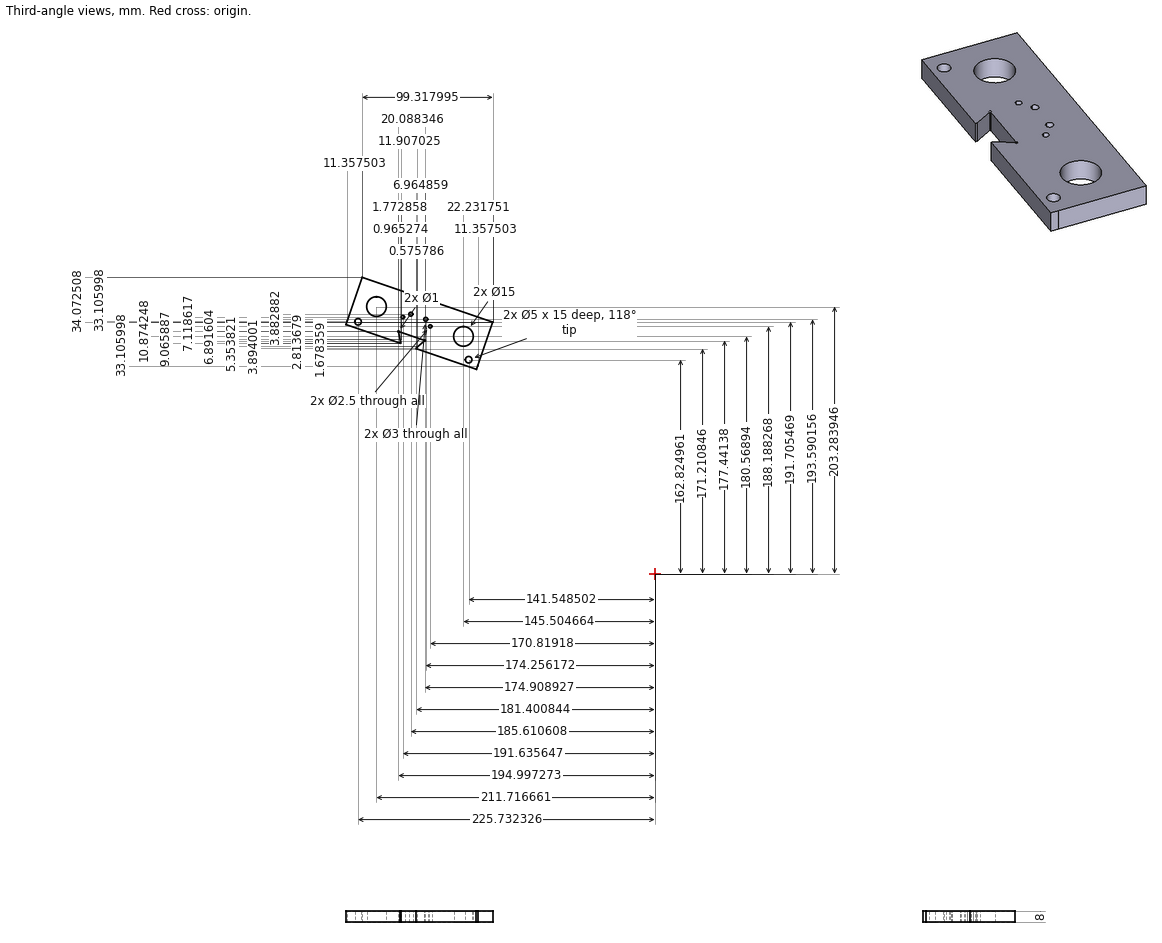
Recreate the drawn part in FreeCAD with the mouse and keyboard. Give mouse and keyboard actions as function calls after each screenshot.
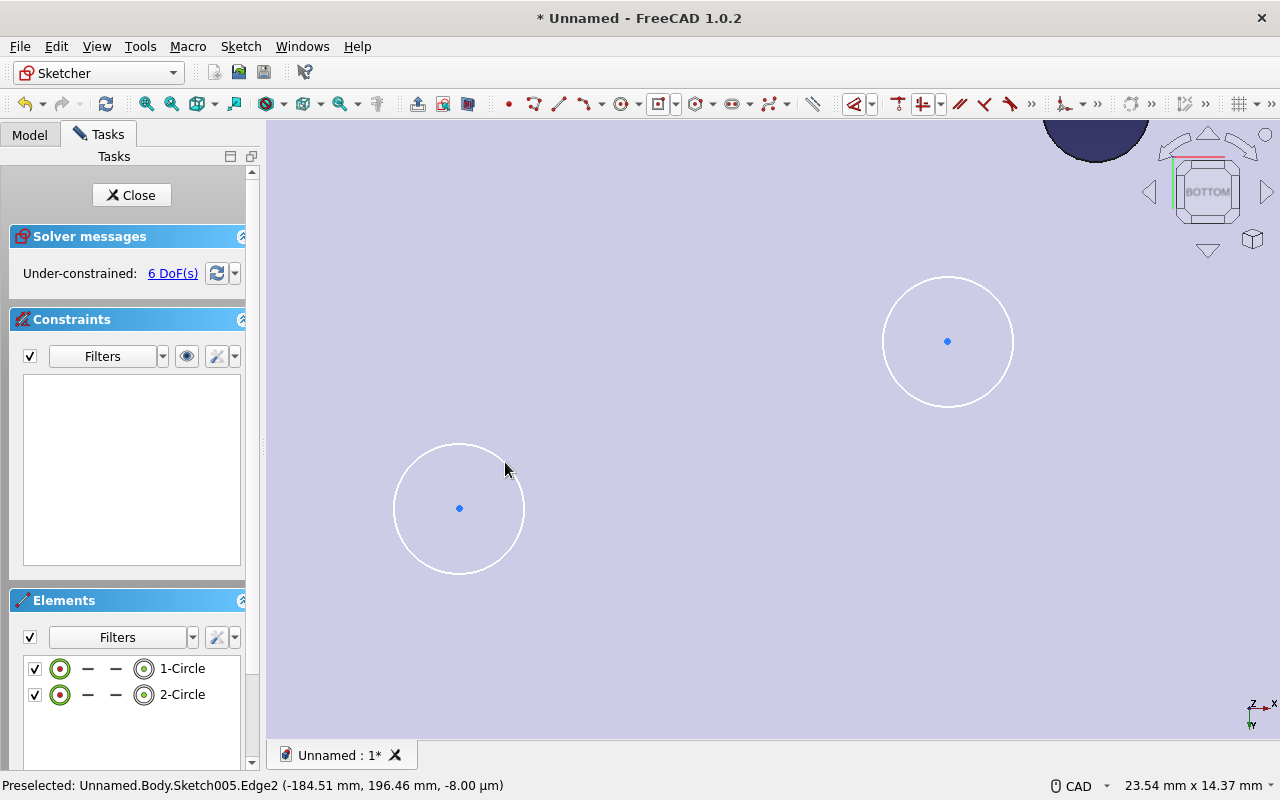
click(994, 296)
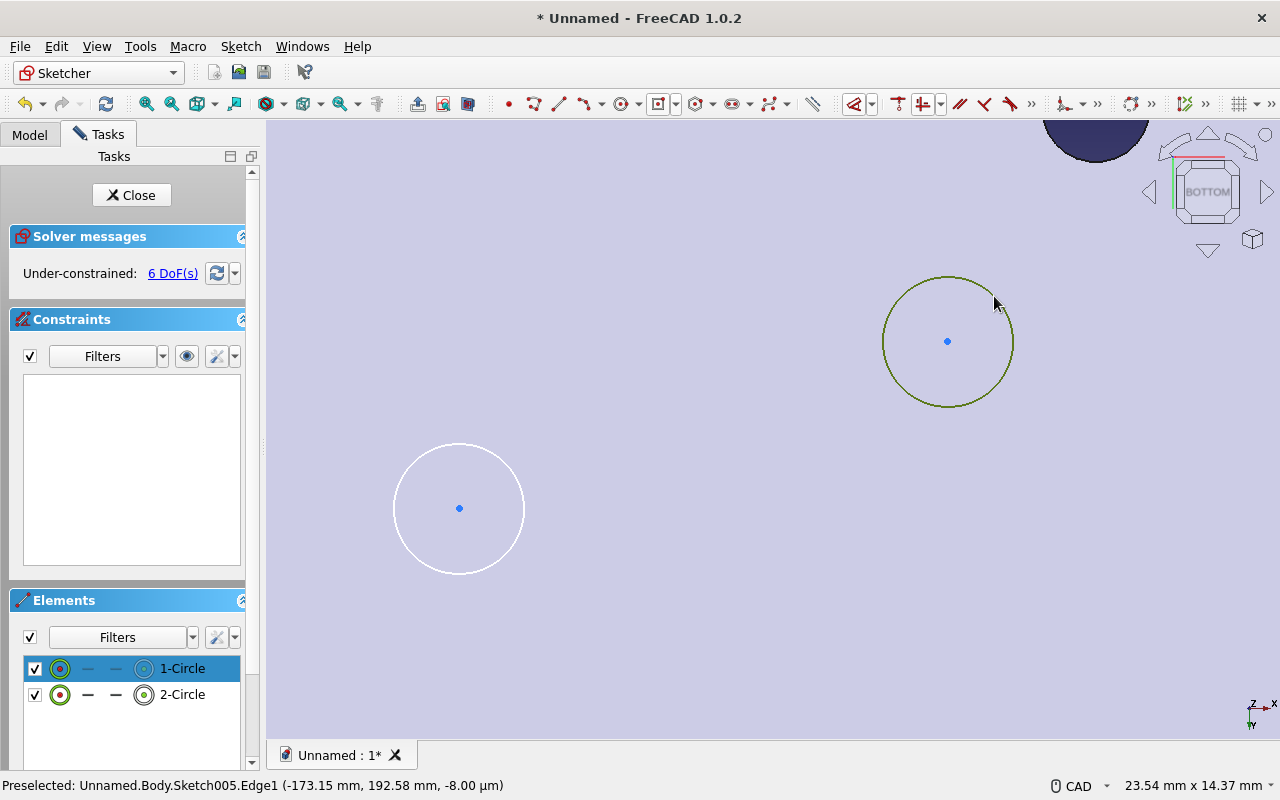
click(505, 463)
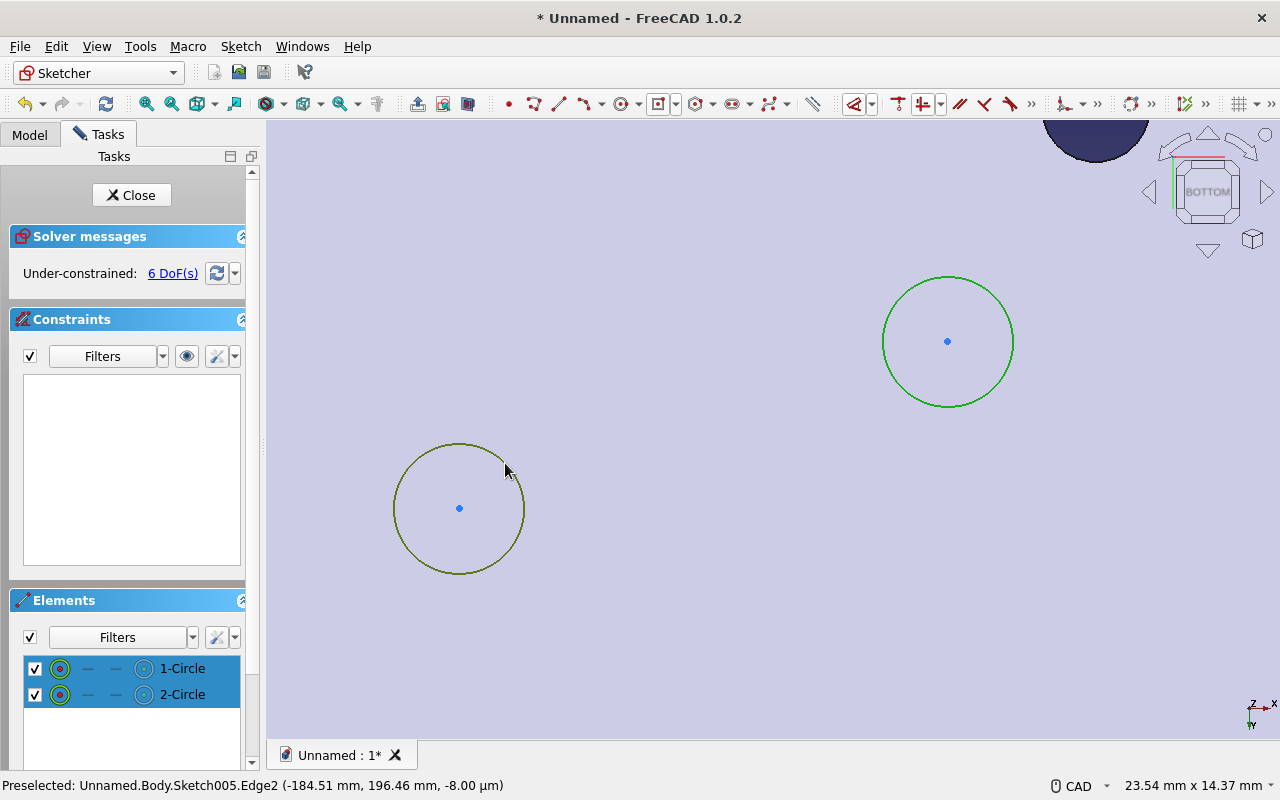
key(e)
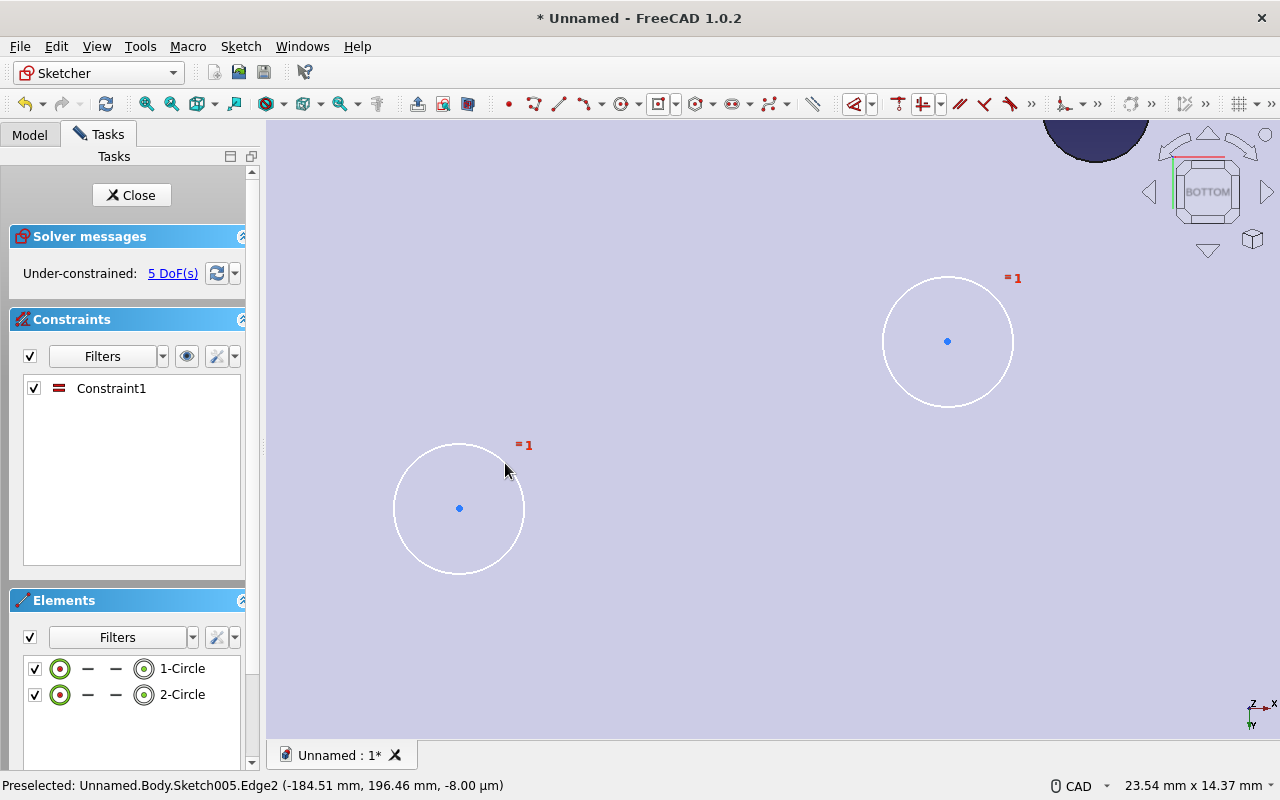
click(994, 296)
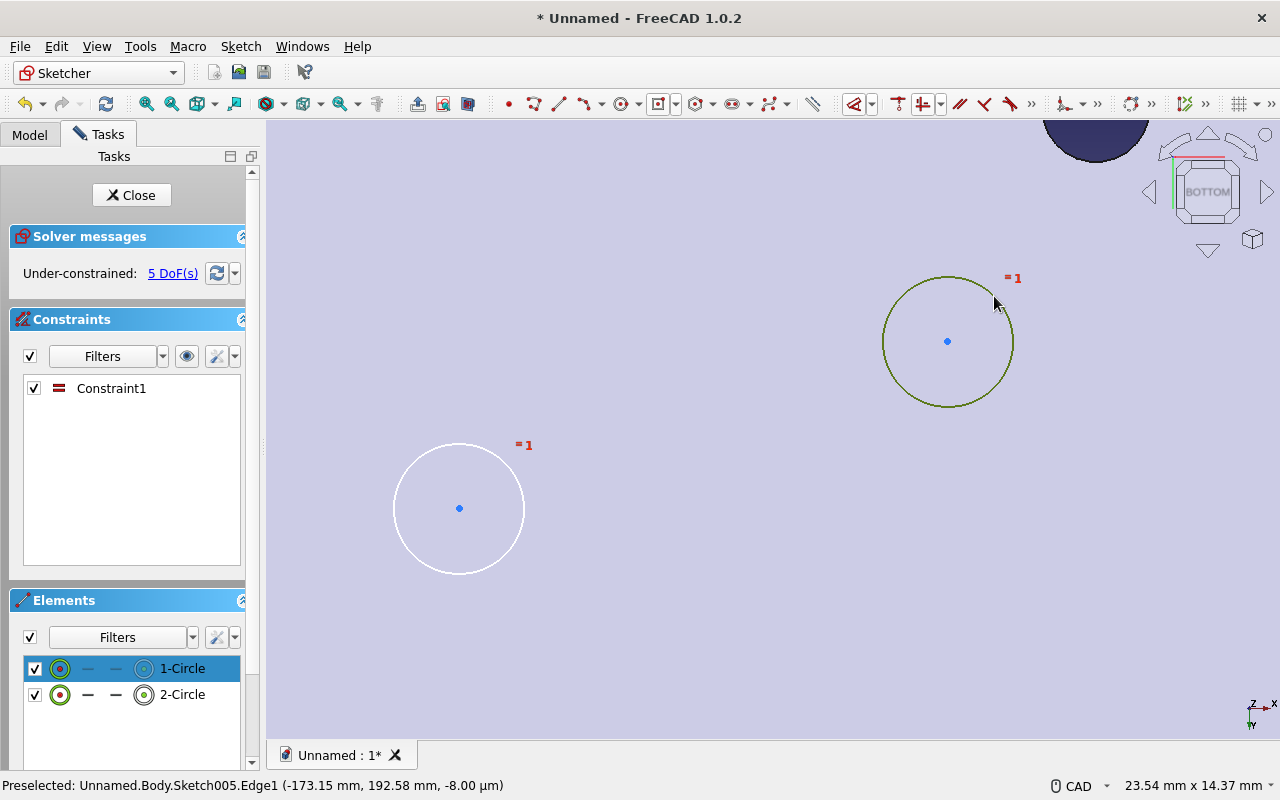
key(k)
key(o)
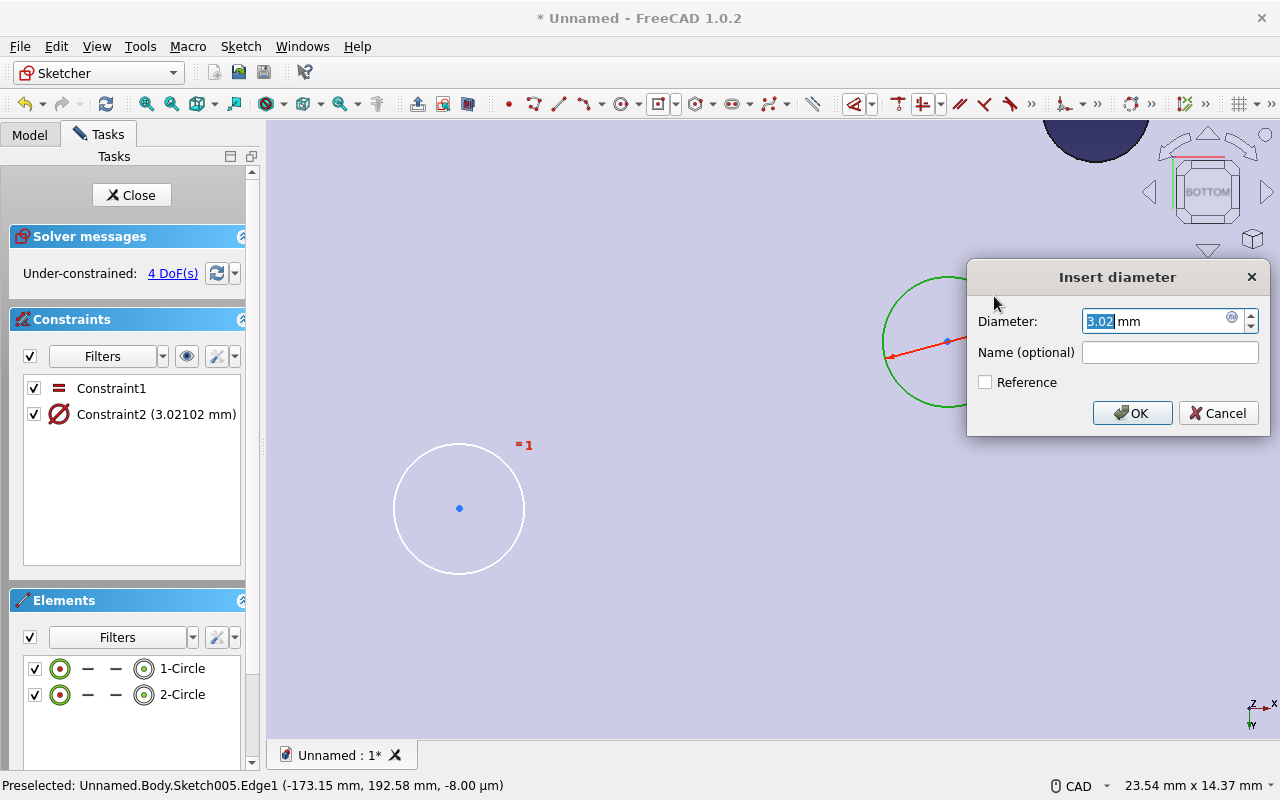
text(3)
key(Return)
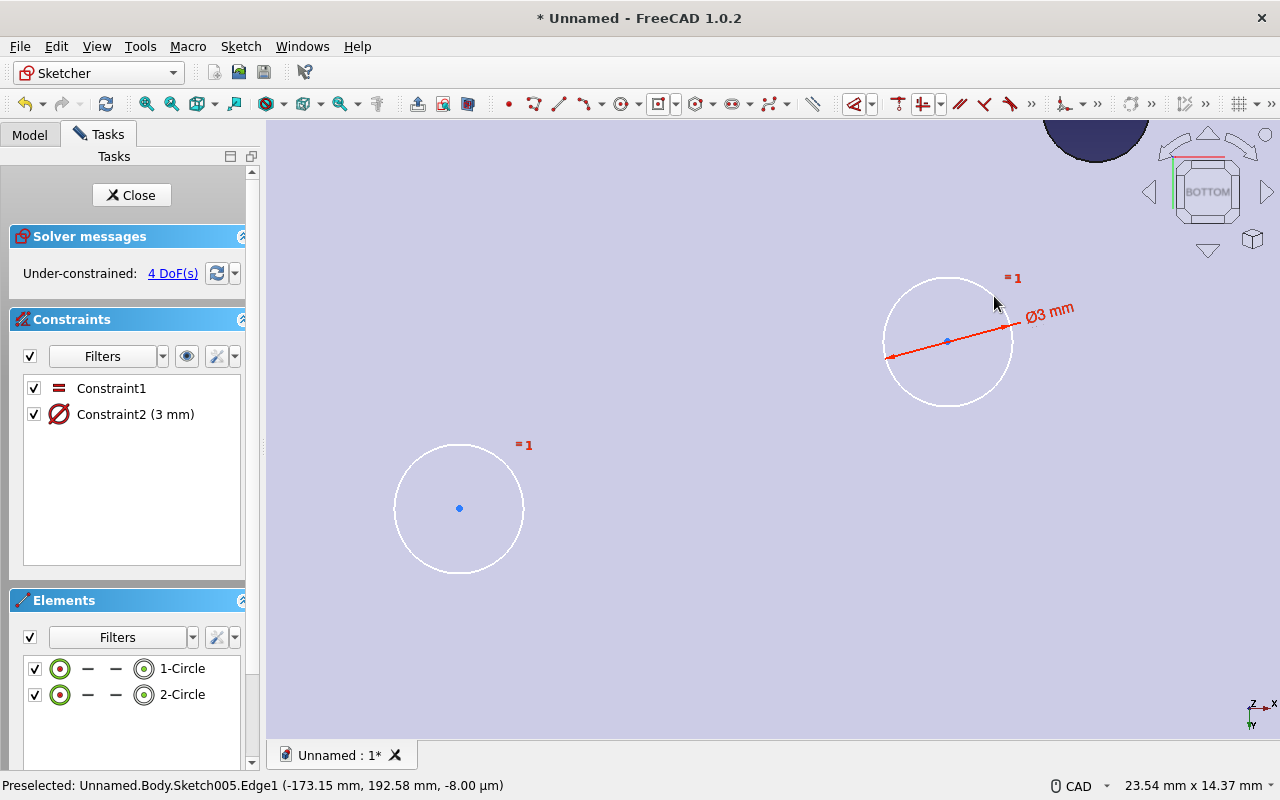
click(948, 342)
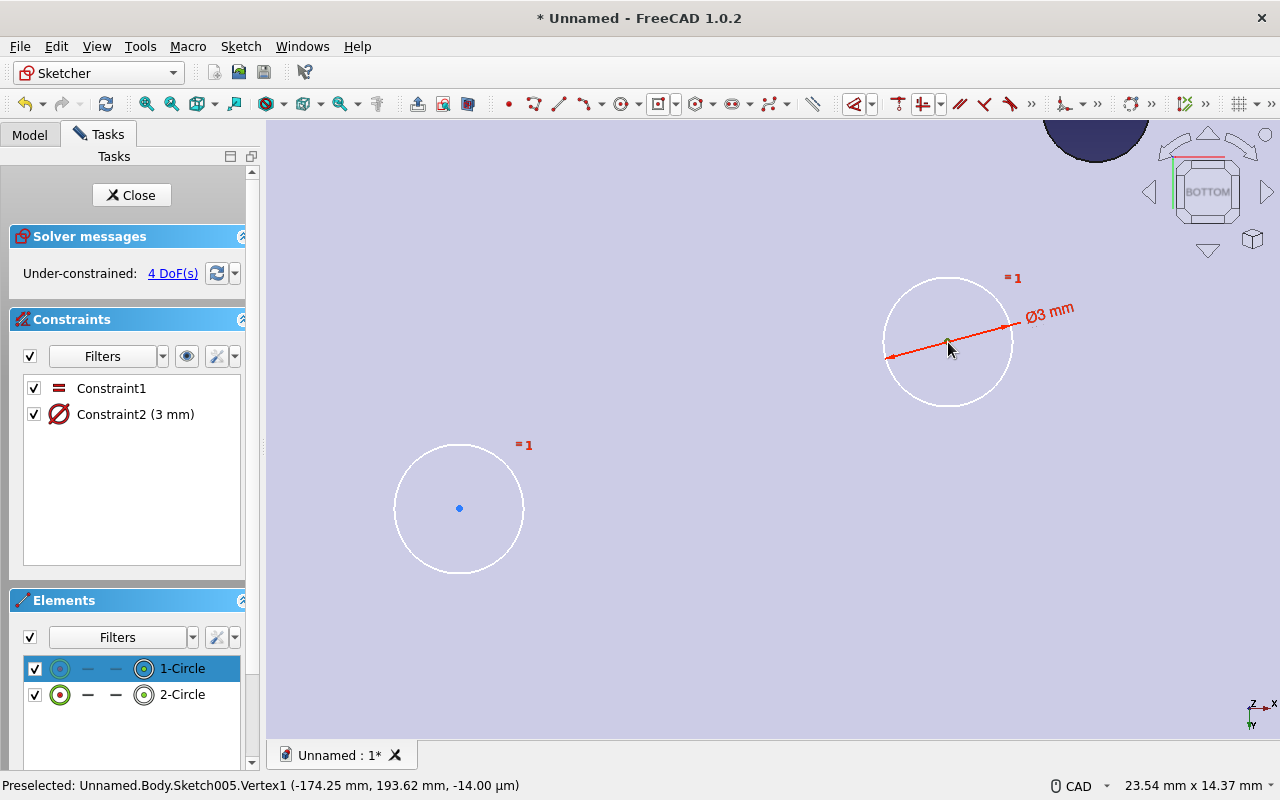
click(459, 509)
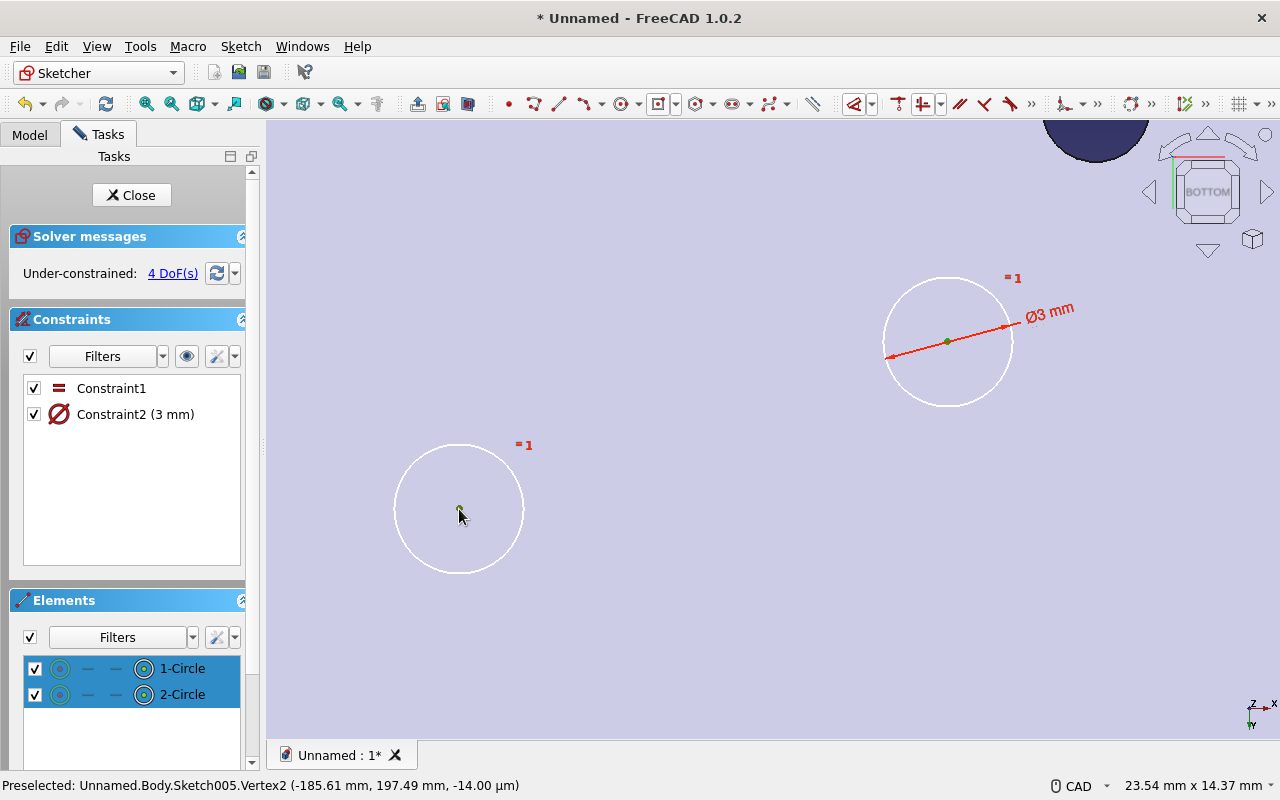
click(872, 104)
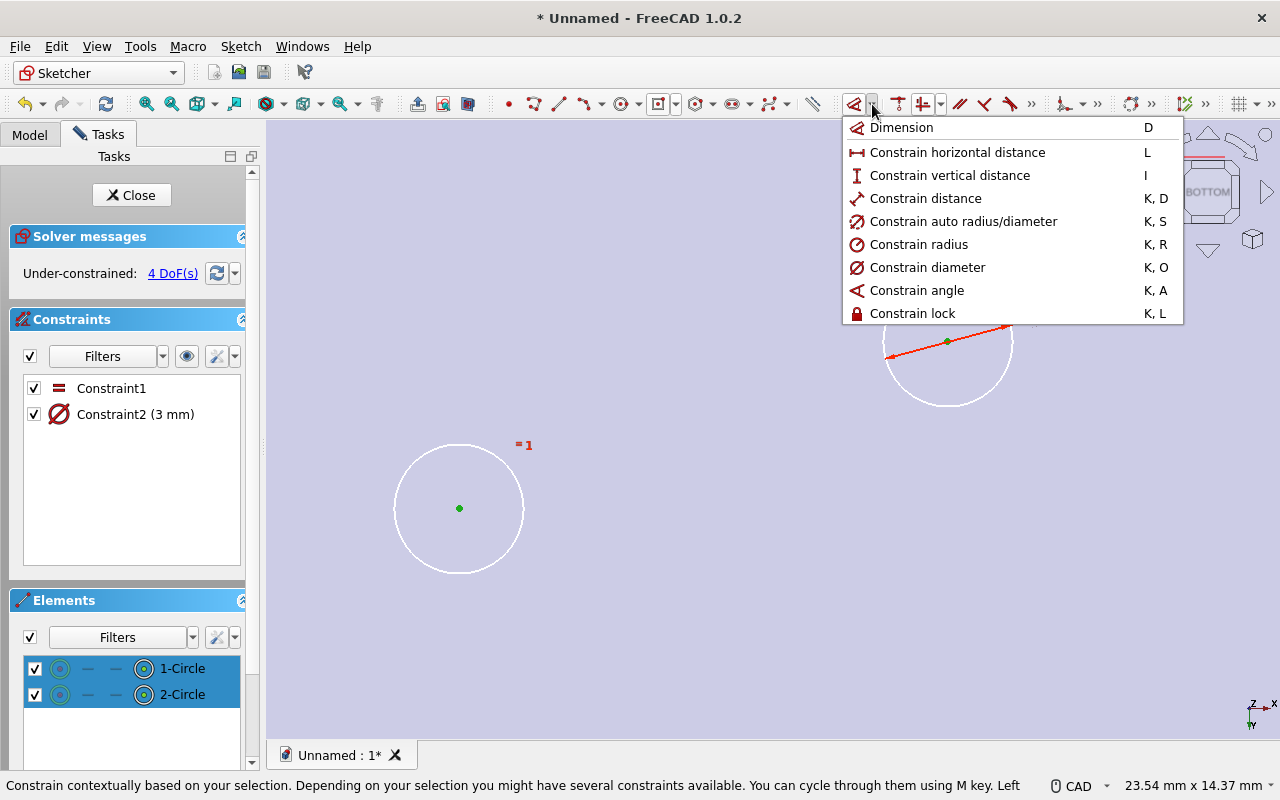
click(1013, 176)